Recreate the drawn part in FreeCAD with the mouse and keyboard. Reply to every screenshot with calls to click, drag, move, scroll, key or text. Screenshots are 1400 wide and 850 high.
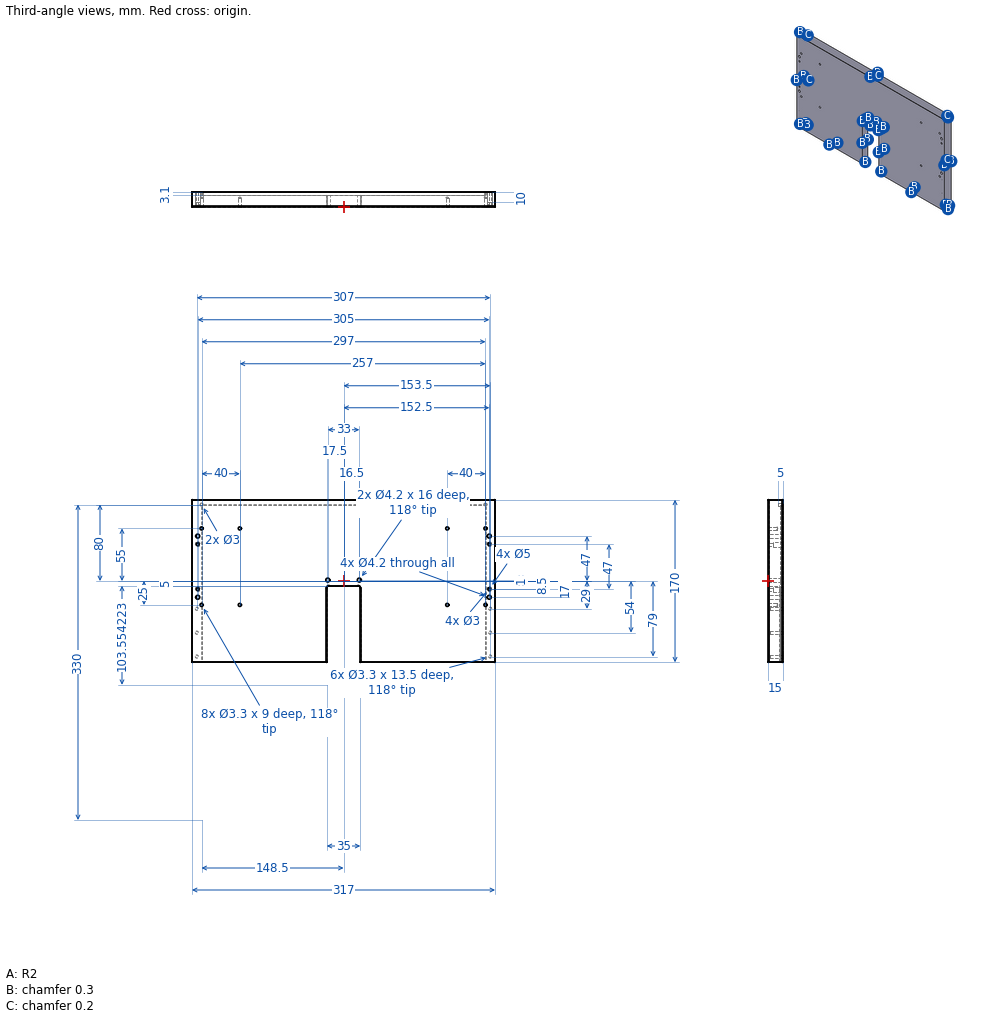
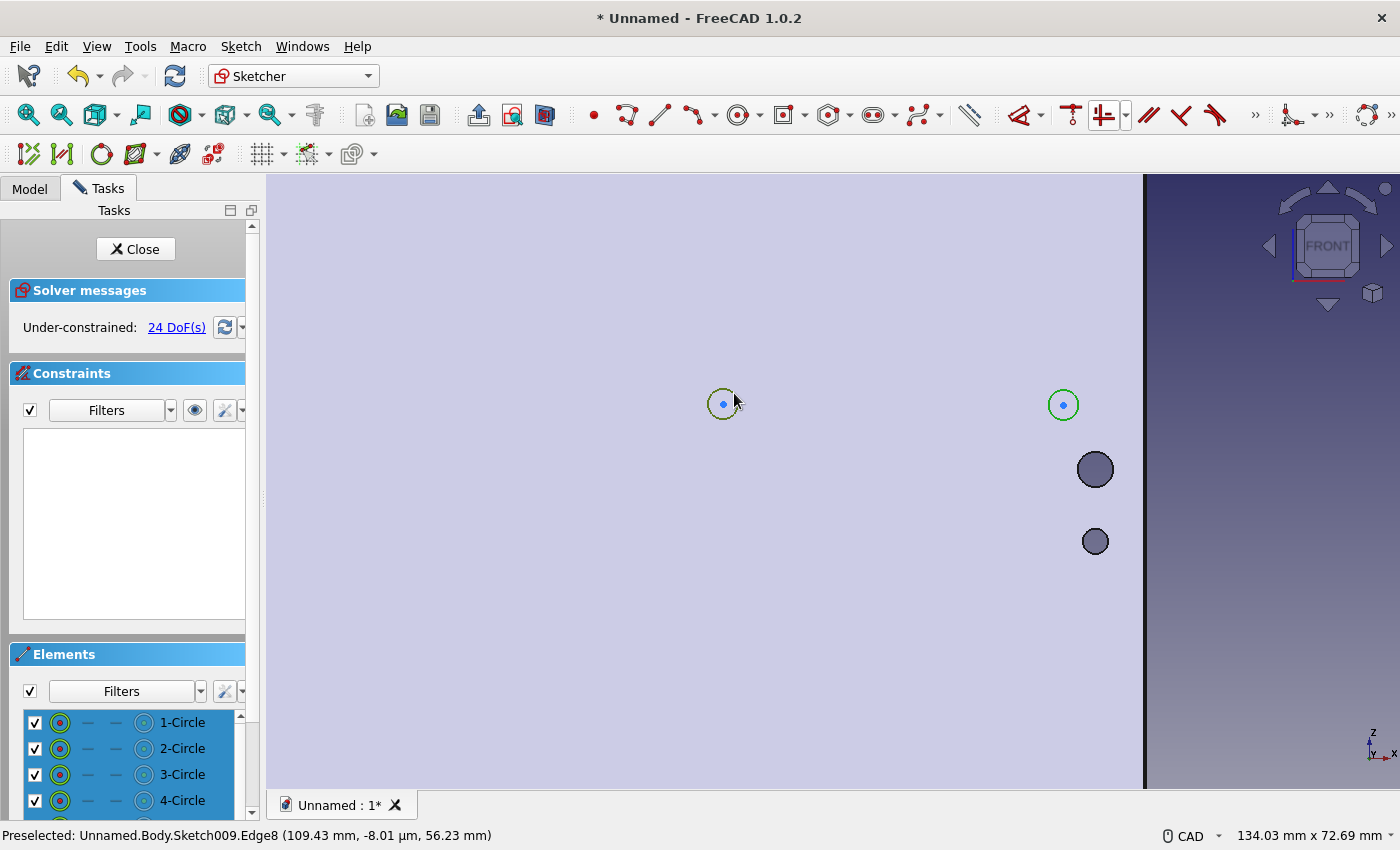
key(e)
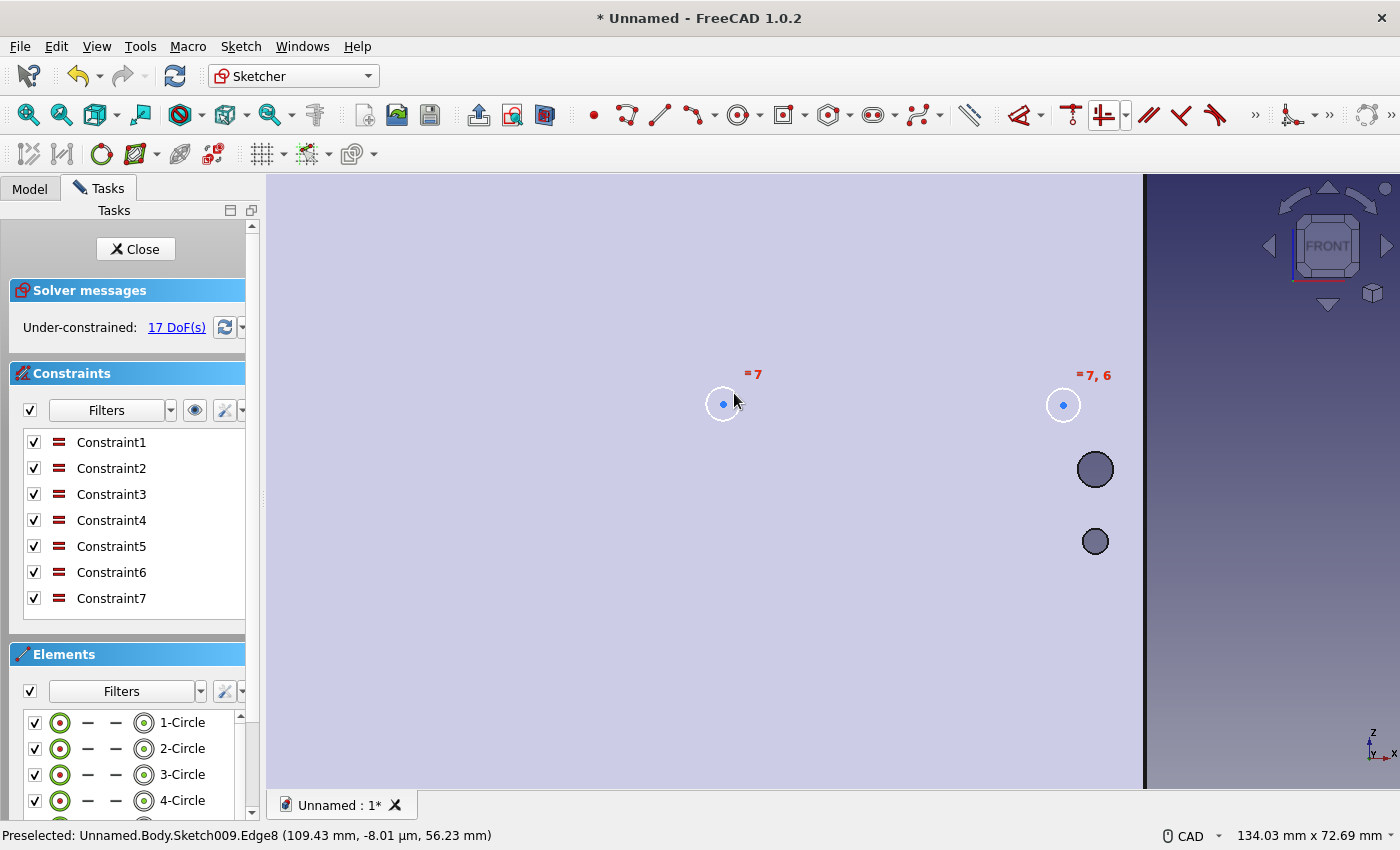
scroll(1079, 397, down, 7)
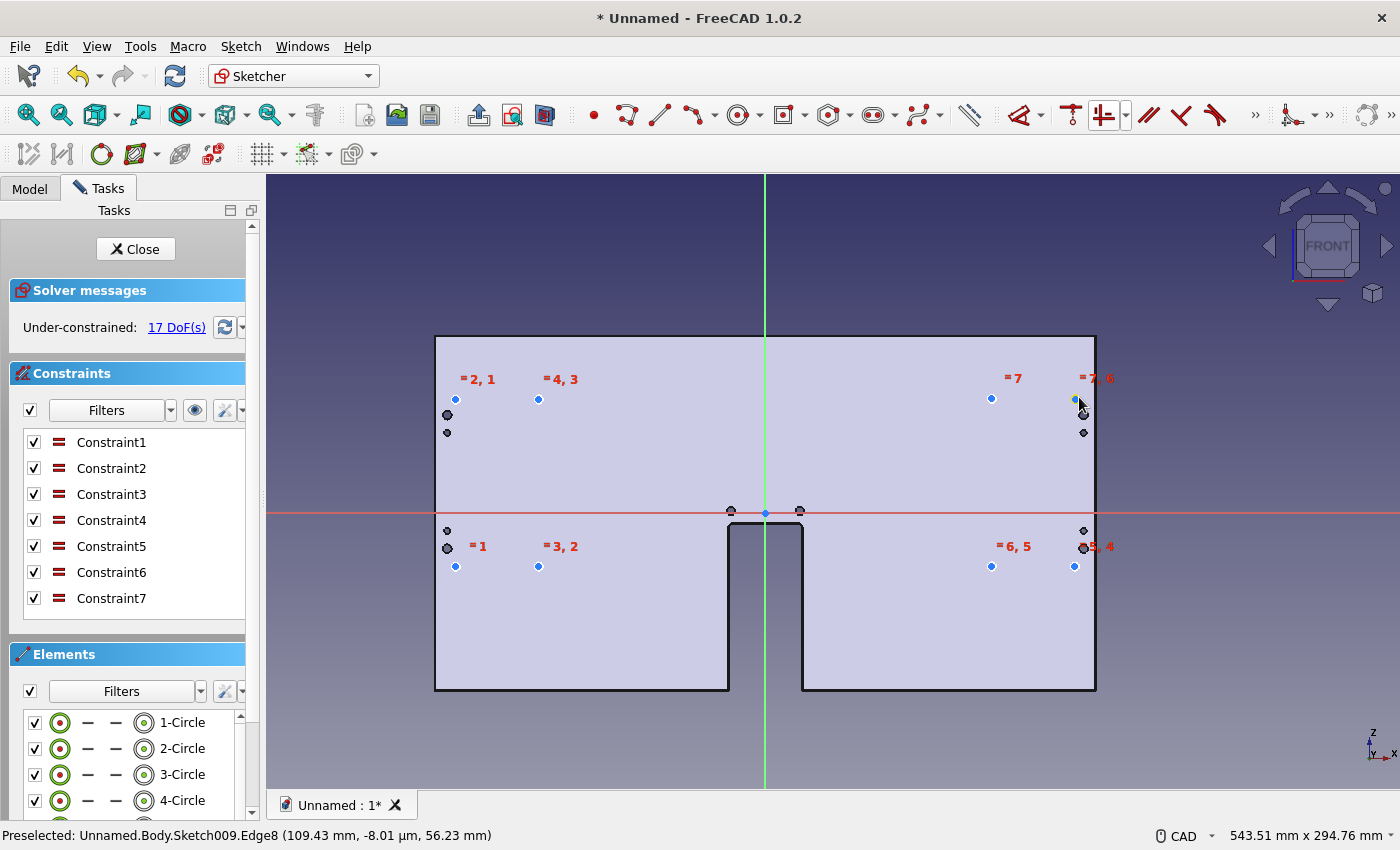
click(456, 567)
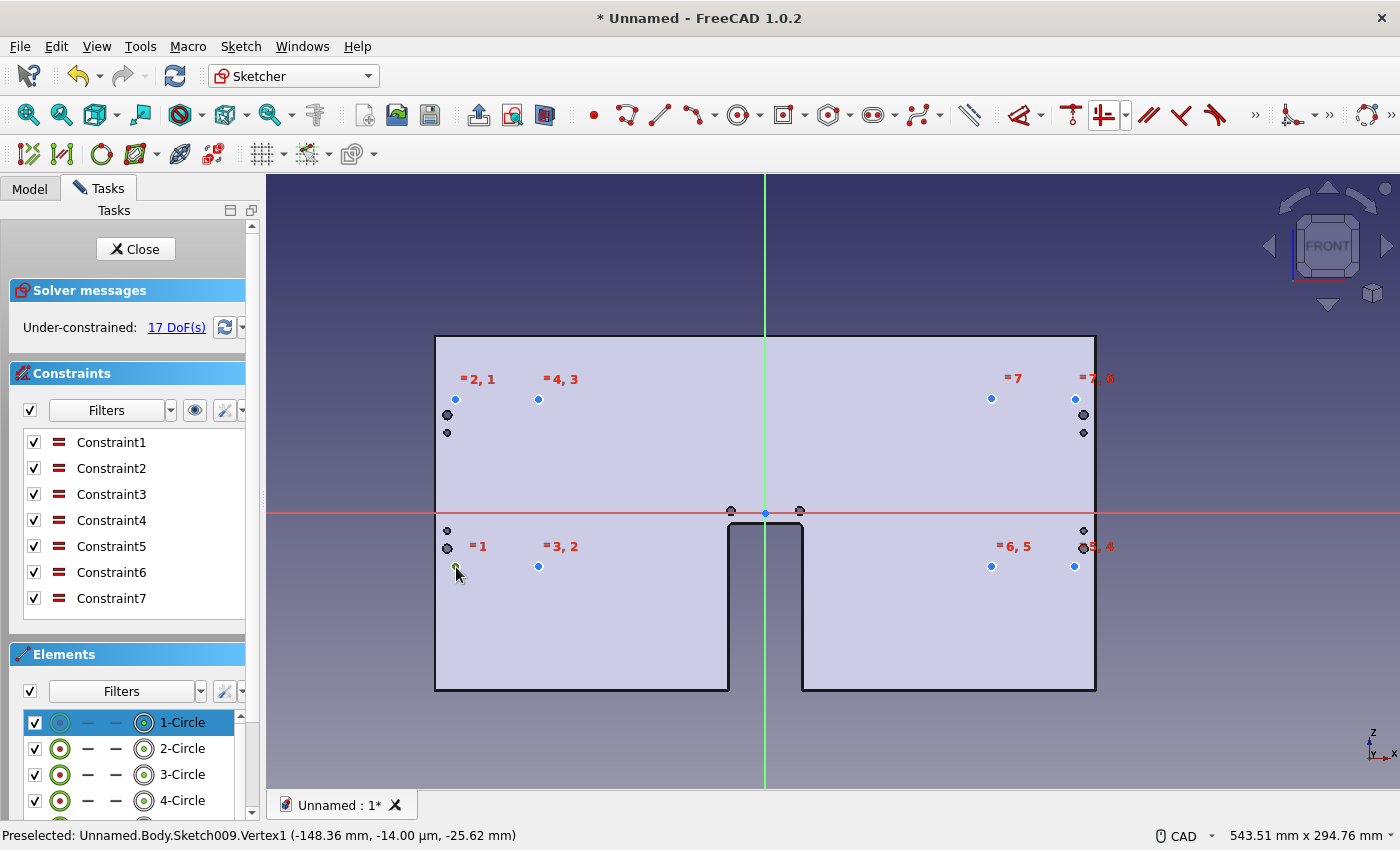
click(456, 400)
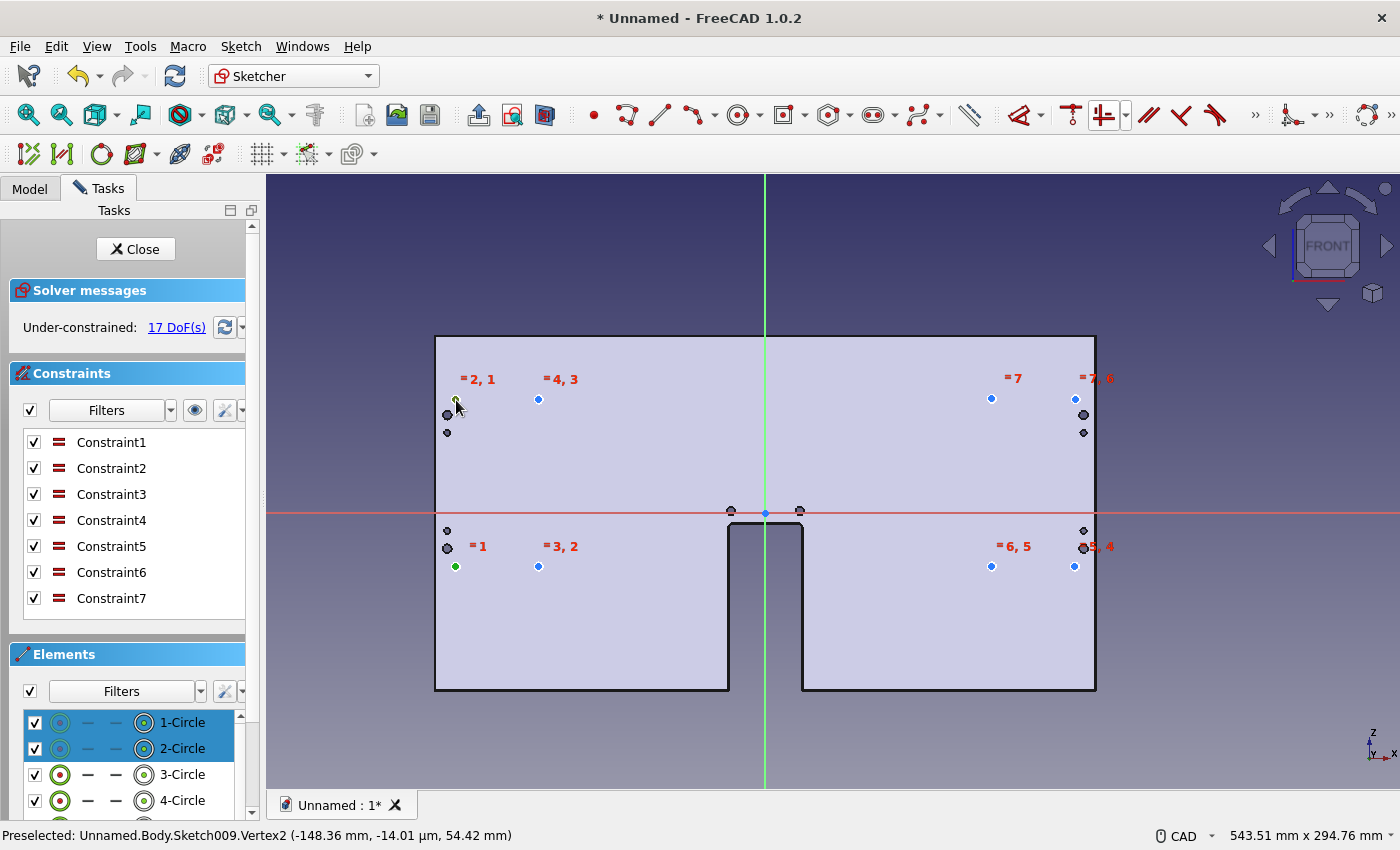
key(v)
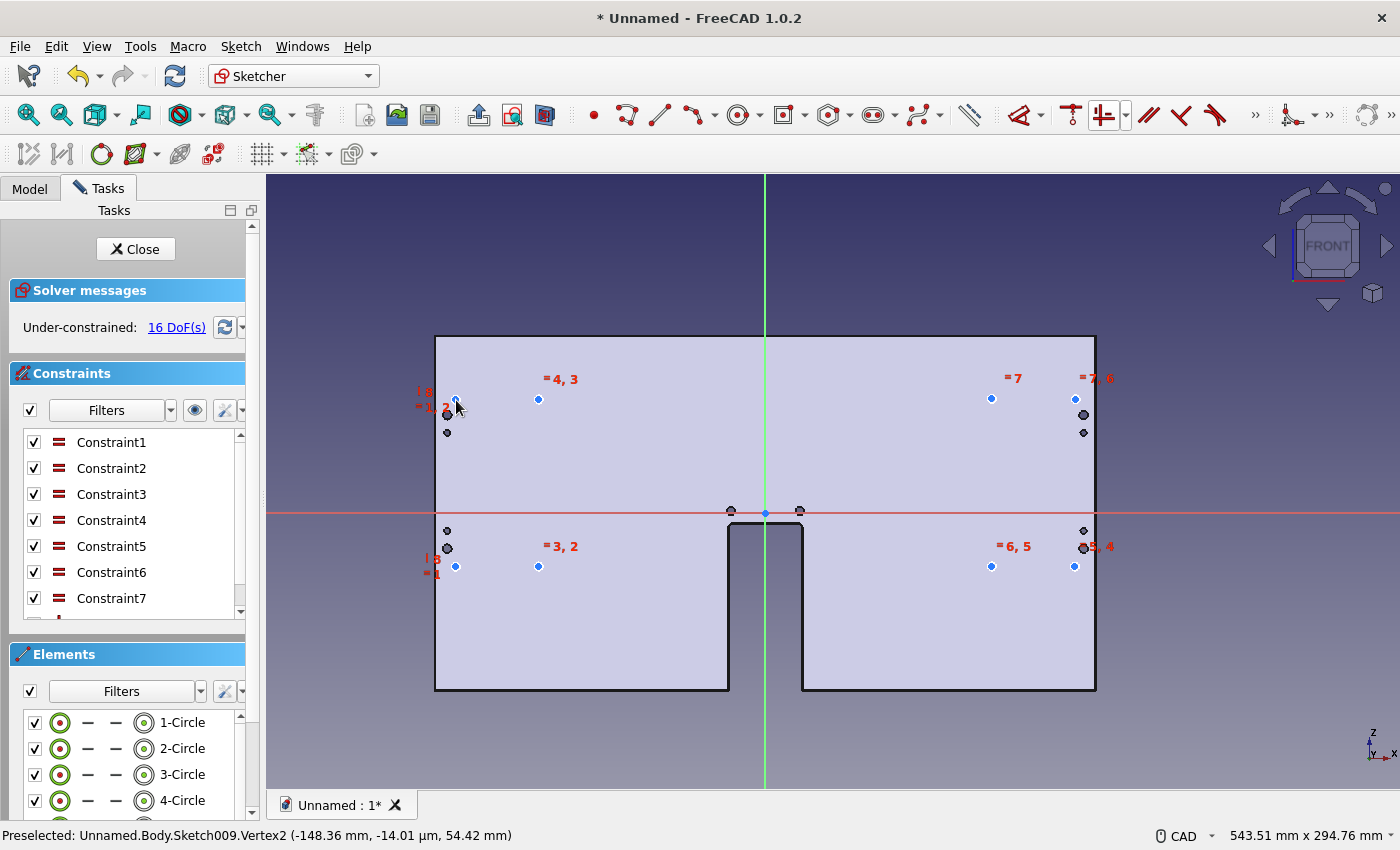
click(456, 567)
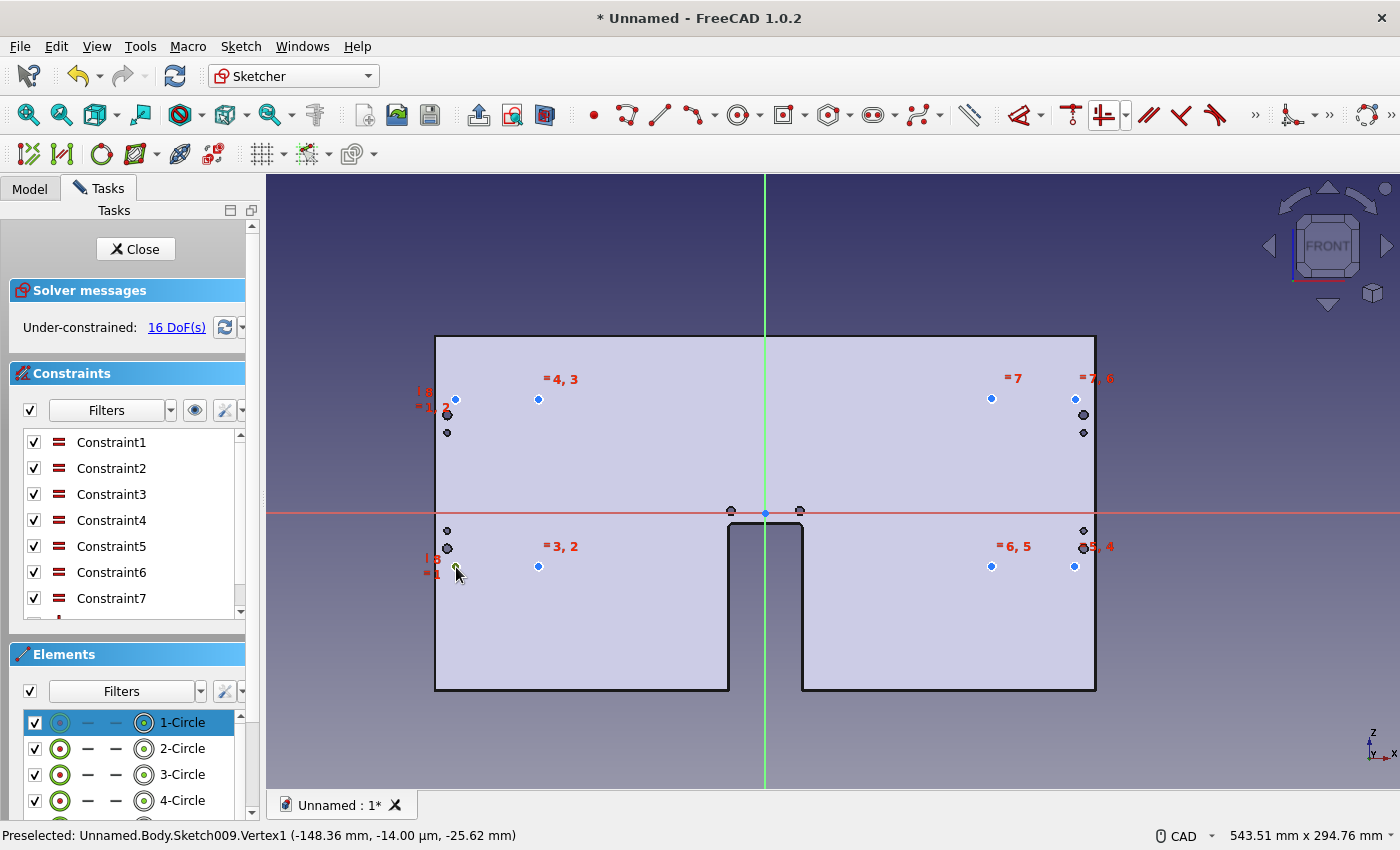
click(539, 567)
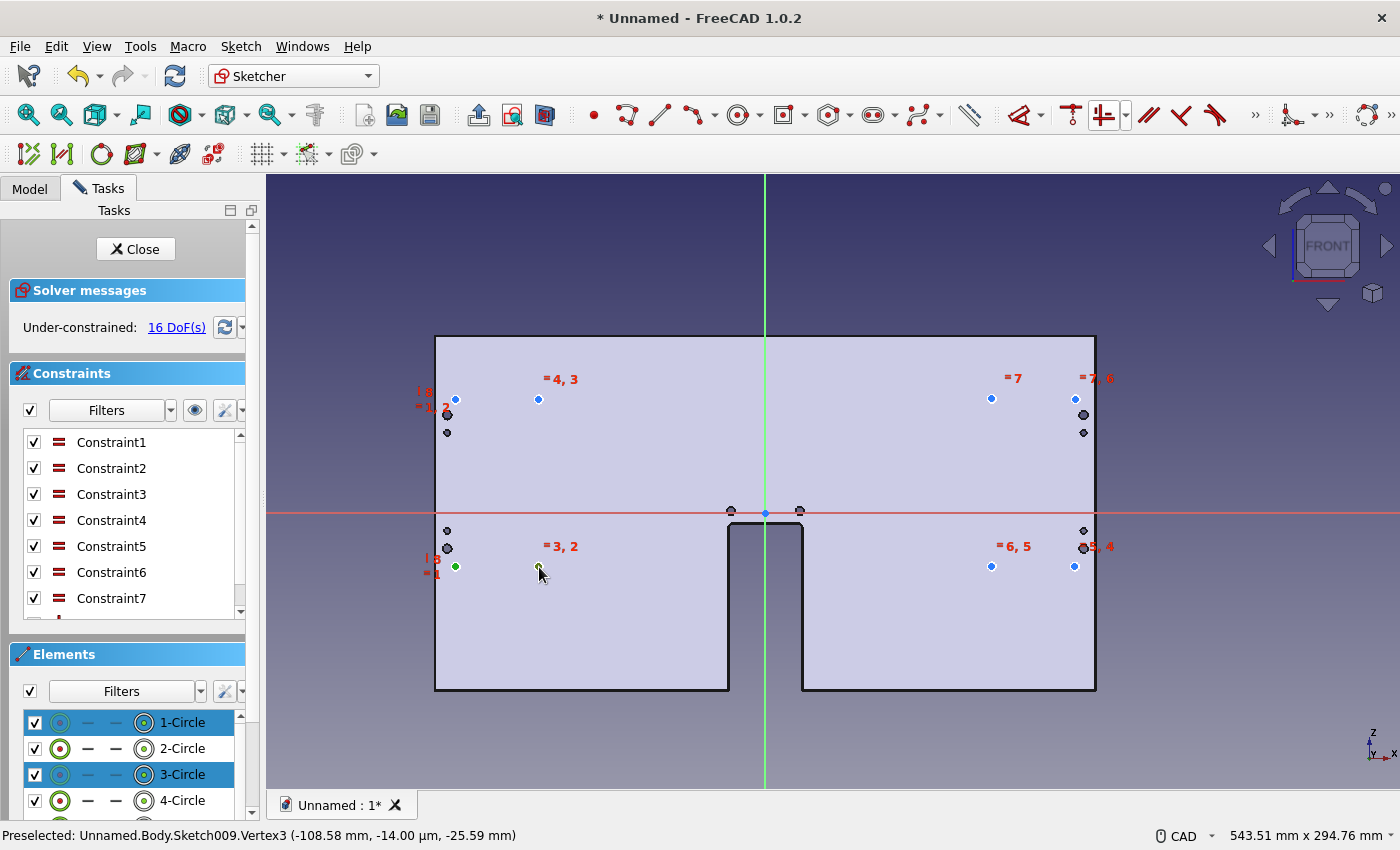
key(h)